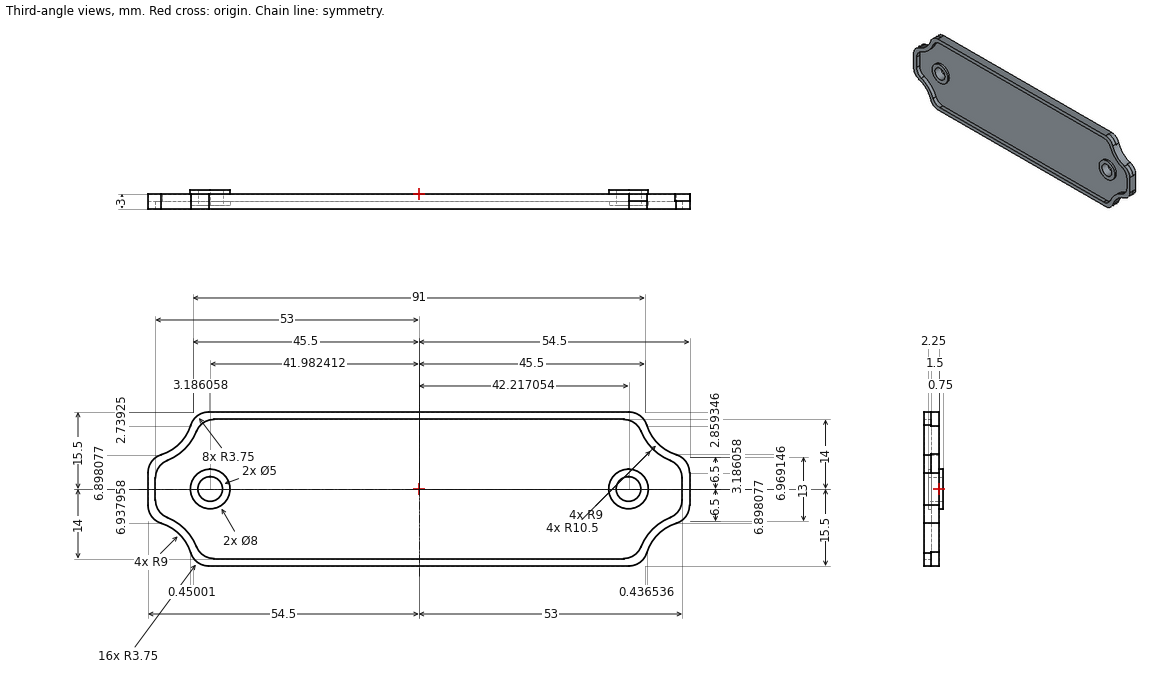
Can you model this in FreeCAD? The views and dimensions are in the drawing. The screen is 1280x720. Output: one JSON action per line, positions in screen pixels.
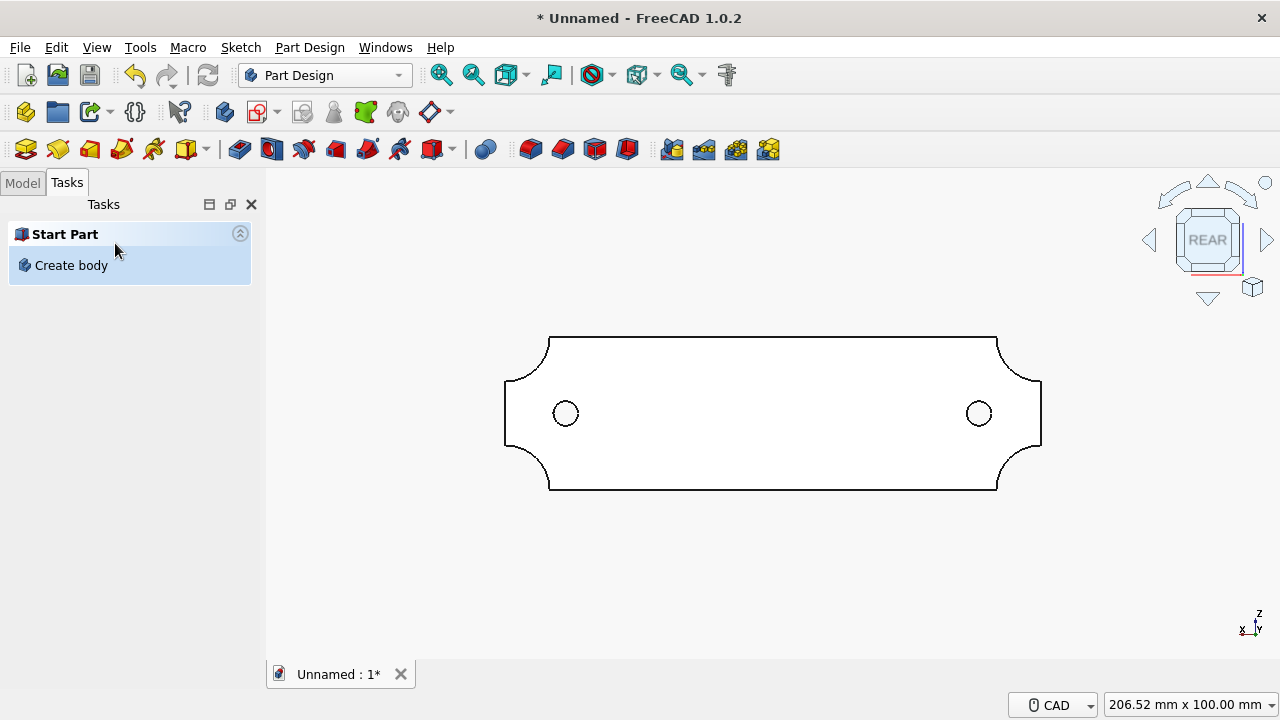
{"action": "left_click", "coordinate": [697, 412]}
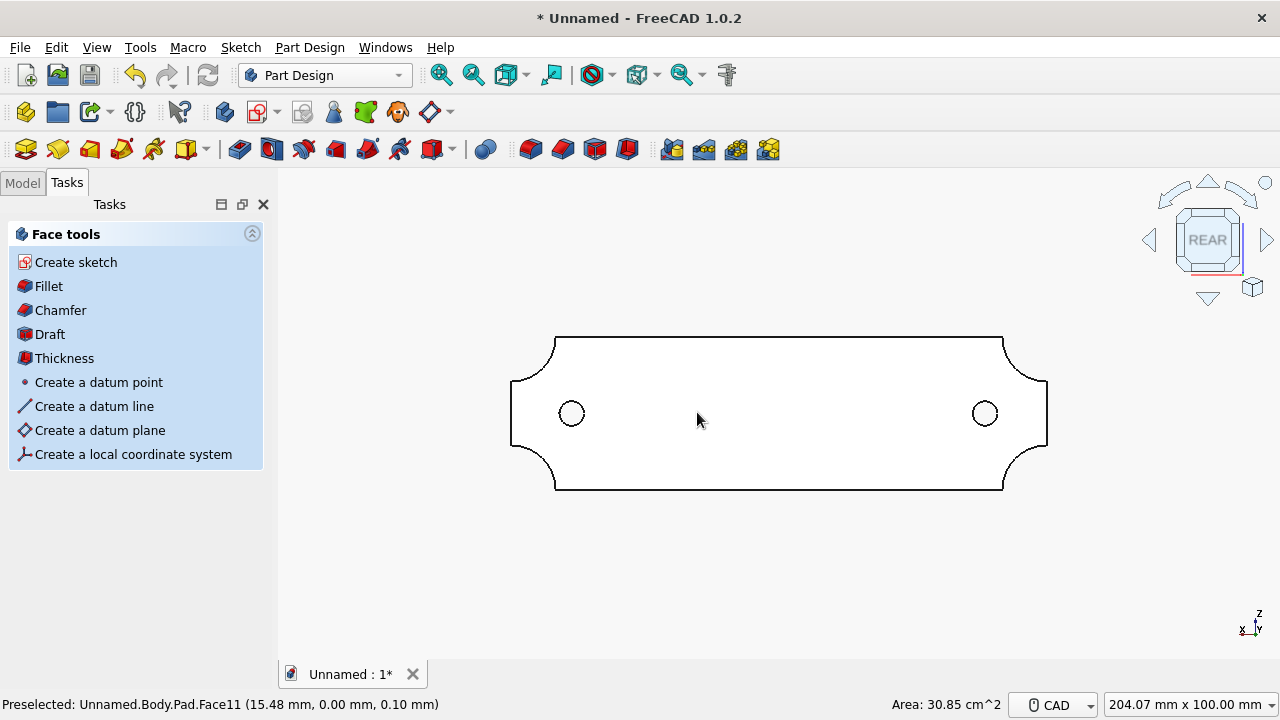
{"action": "left_click", "coordinate": [258, 112]}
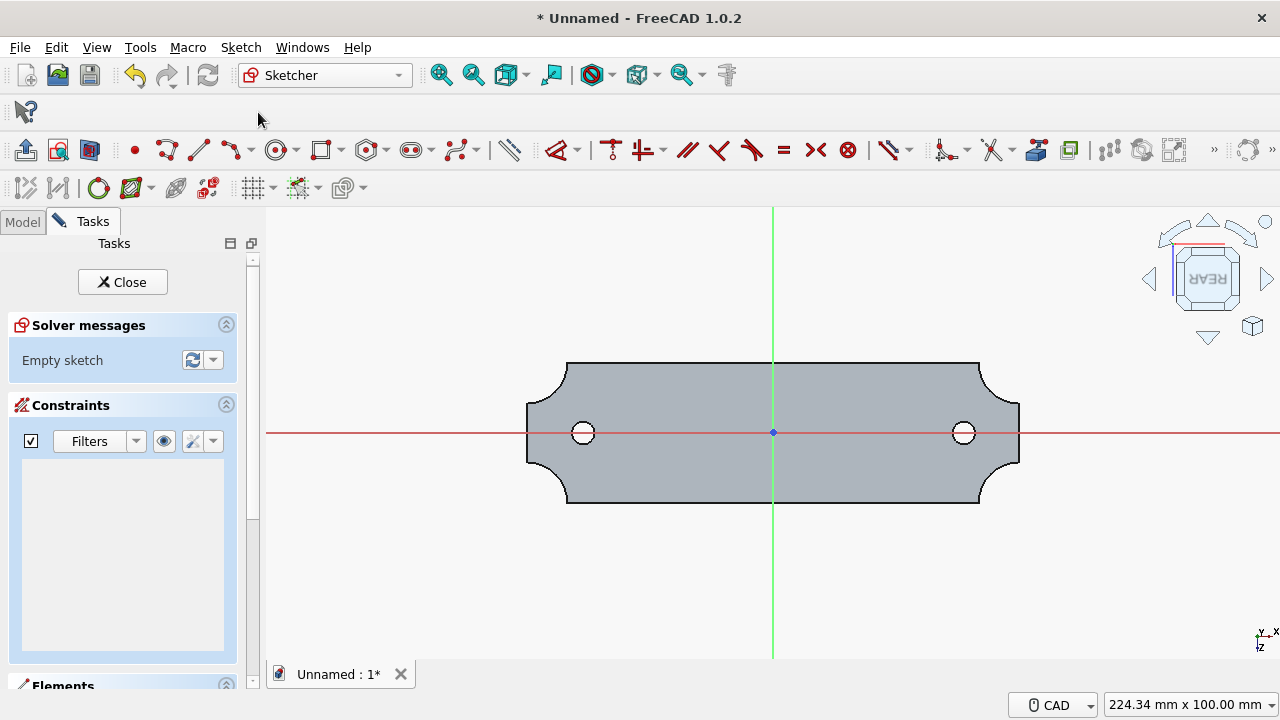
{"action": "left_click", "coordinate": [200, 150]}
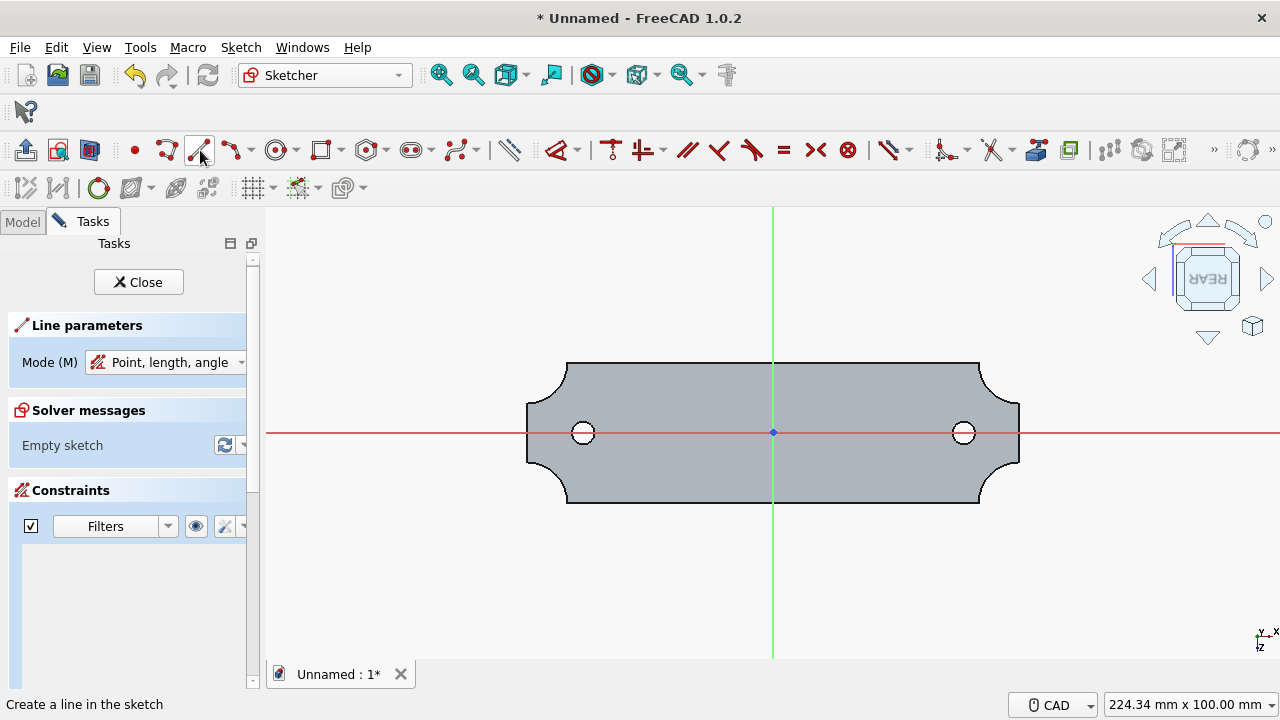
{"action": "left_click", "coordinate": [964, 363]}
{"action": "left_click", "coordinate": [582, 363]}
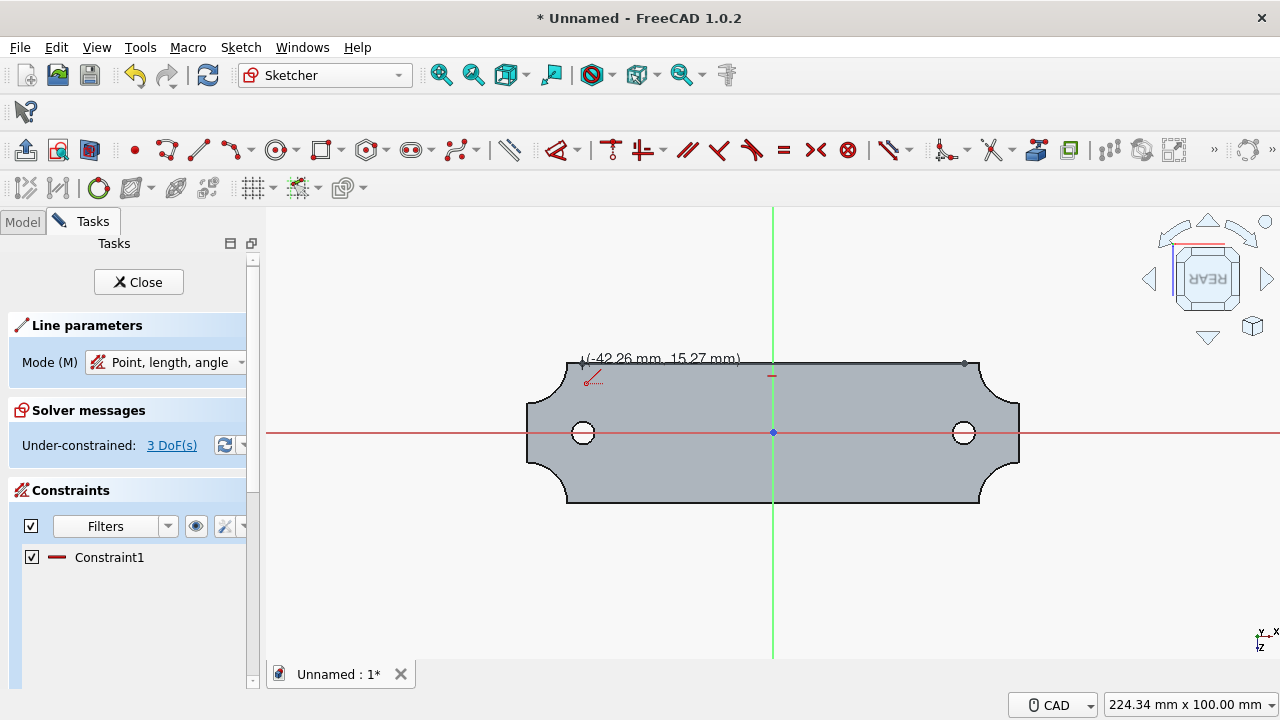
{"action": "left_click", "coordinate": [527, 418]}
{"action": "left_click", "coordinate": [527, 448]}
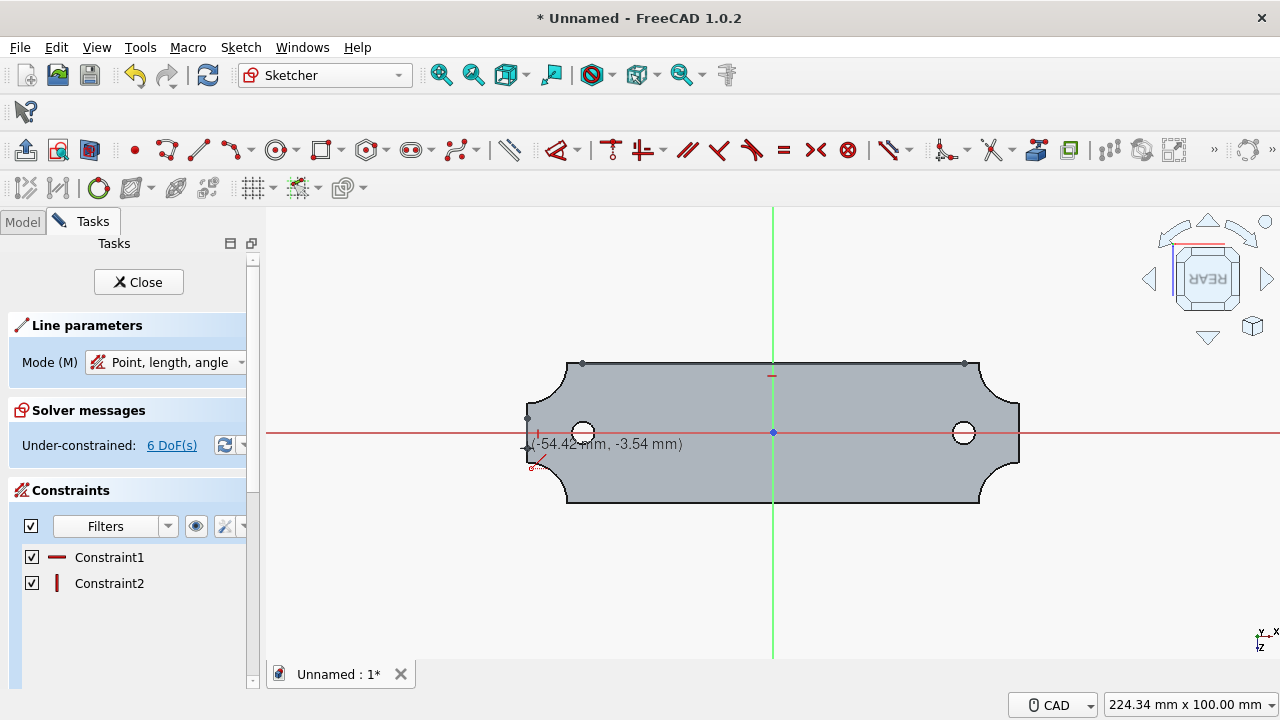
{"action": "left_click", "coordinate": [582, 503]}
{"action": "left_click", "coordinate": [964, 503]}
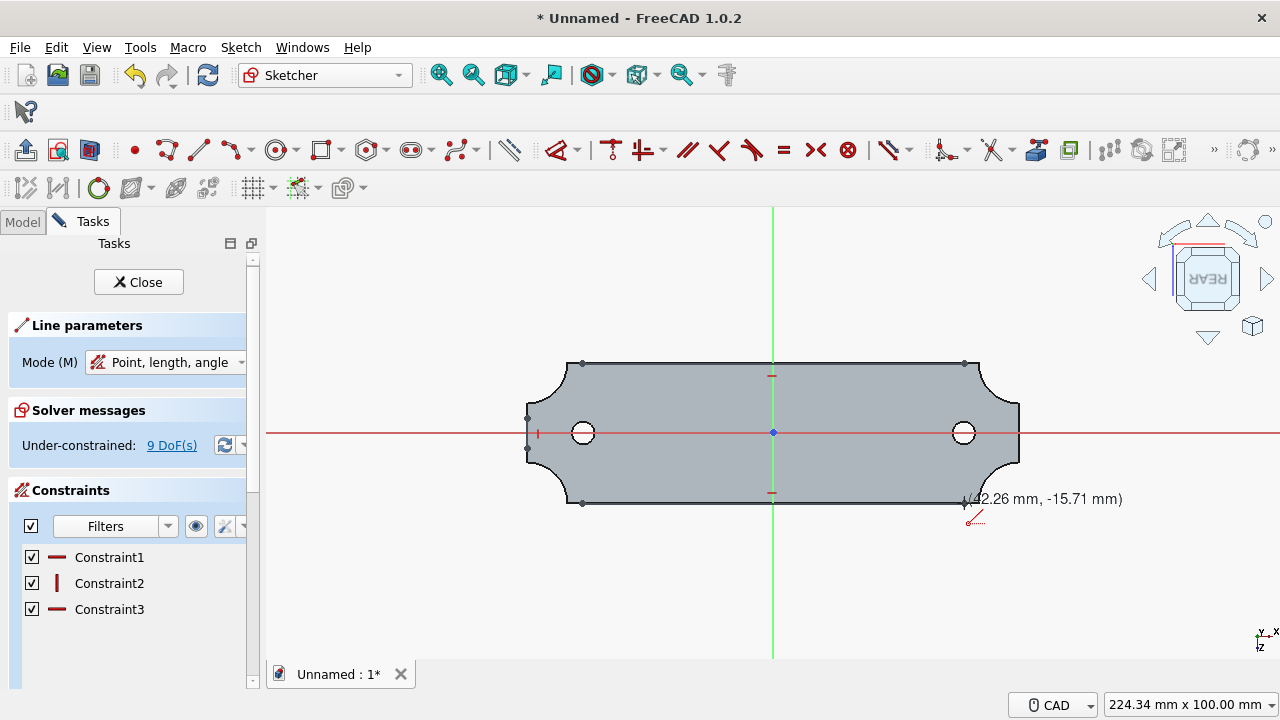
{"action": "left_click", "coordinate": [1019, 448]}
{"action": "left_click", "coordinate": [1019, 418]}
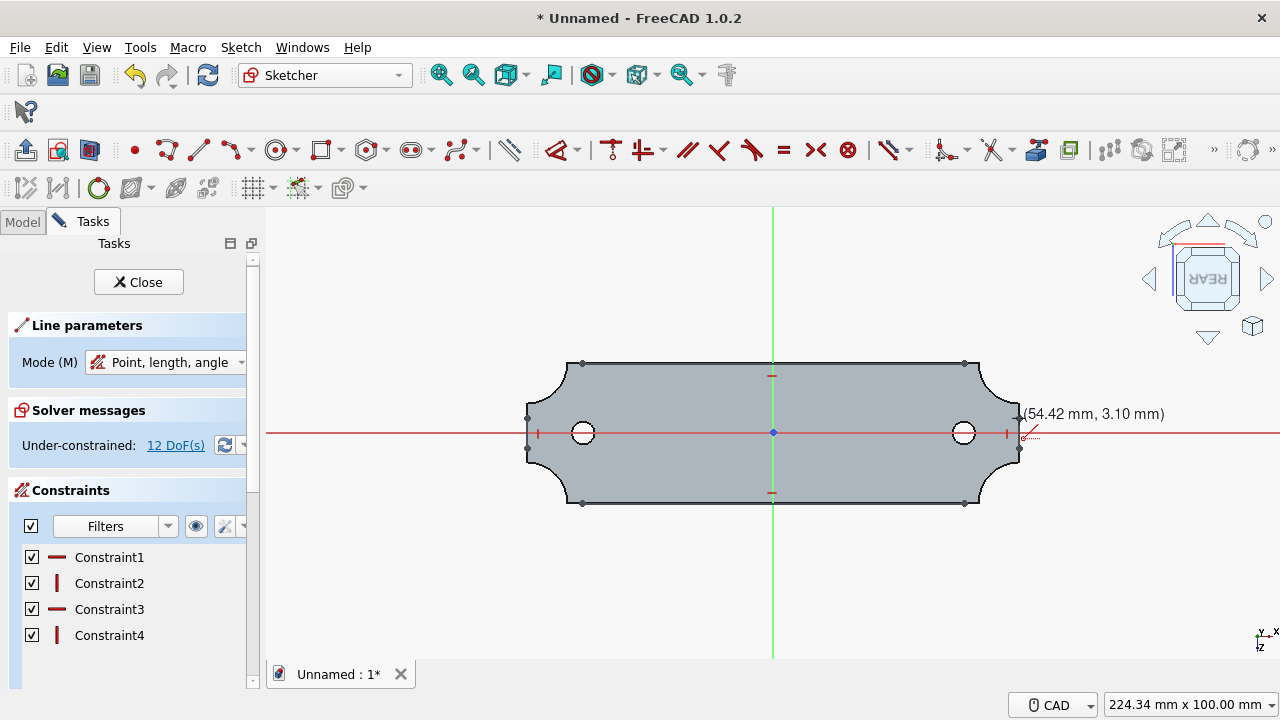
{"action": "left_click", "coordinate": [232, 150]}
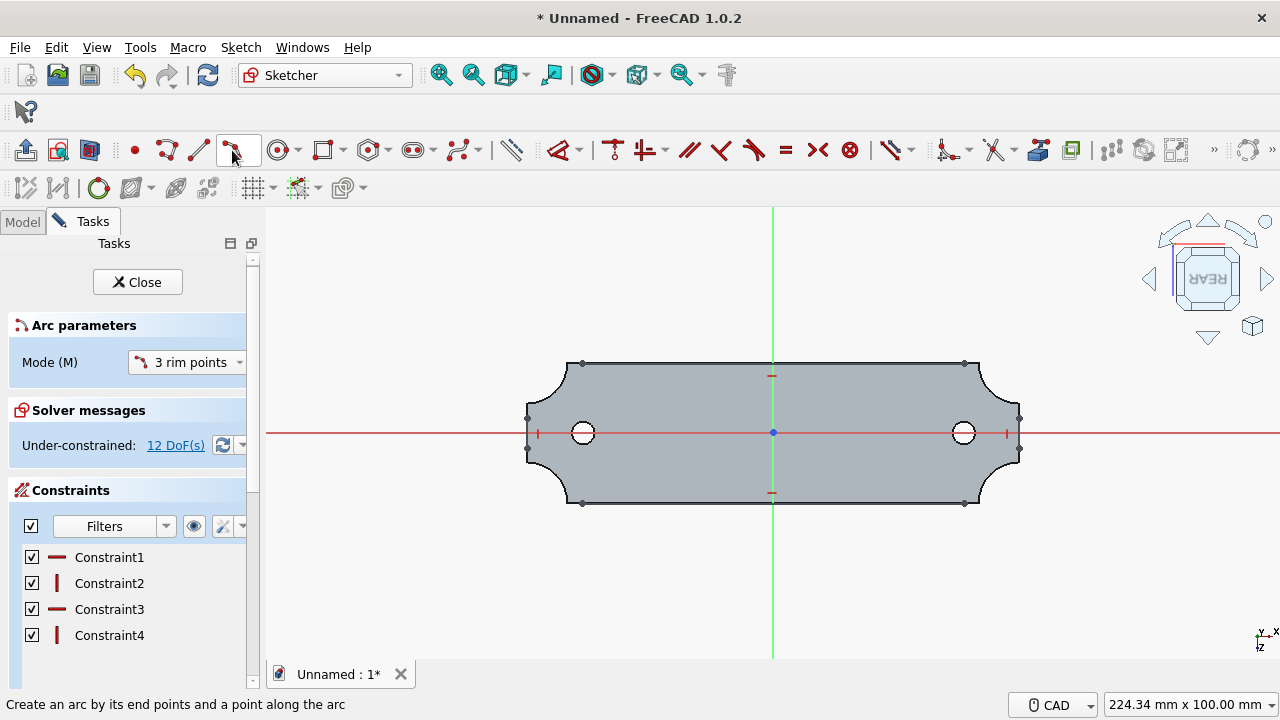
{"action": "left_click", "coordinate": [582, 364]}
{"action": "left_click", "coordinate": [566, 375]}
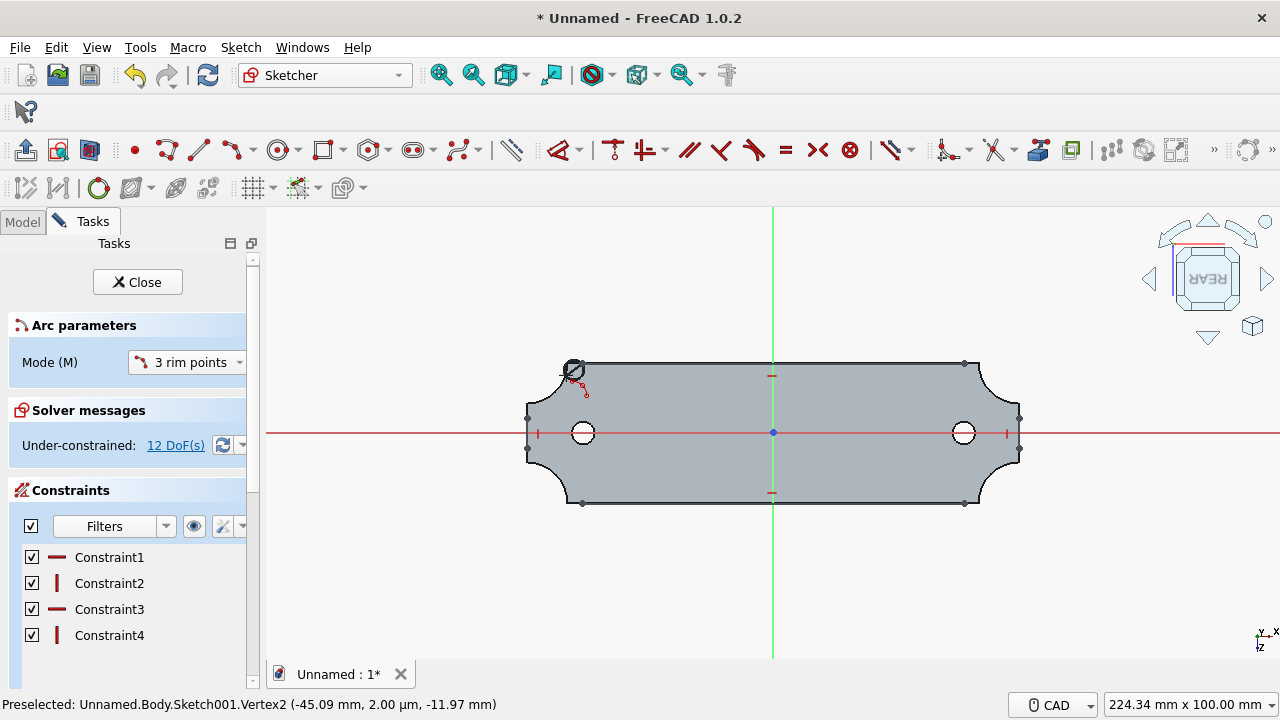
{"action": "scroll", "coordinate": [572, 366], "scroll_direction": "up", "scroll_amount": 8}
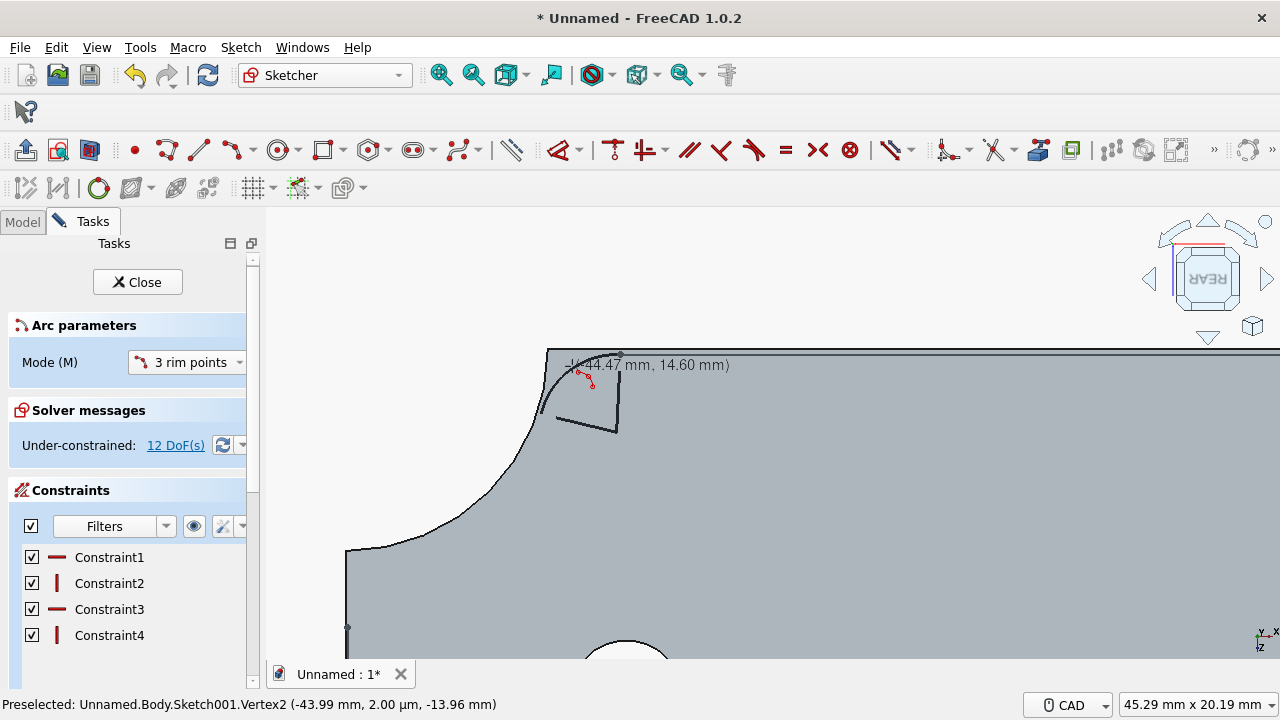
{"action": "left_click", "coordinate": [569, 366]}